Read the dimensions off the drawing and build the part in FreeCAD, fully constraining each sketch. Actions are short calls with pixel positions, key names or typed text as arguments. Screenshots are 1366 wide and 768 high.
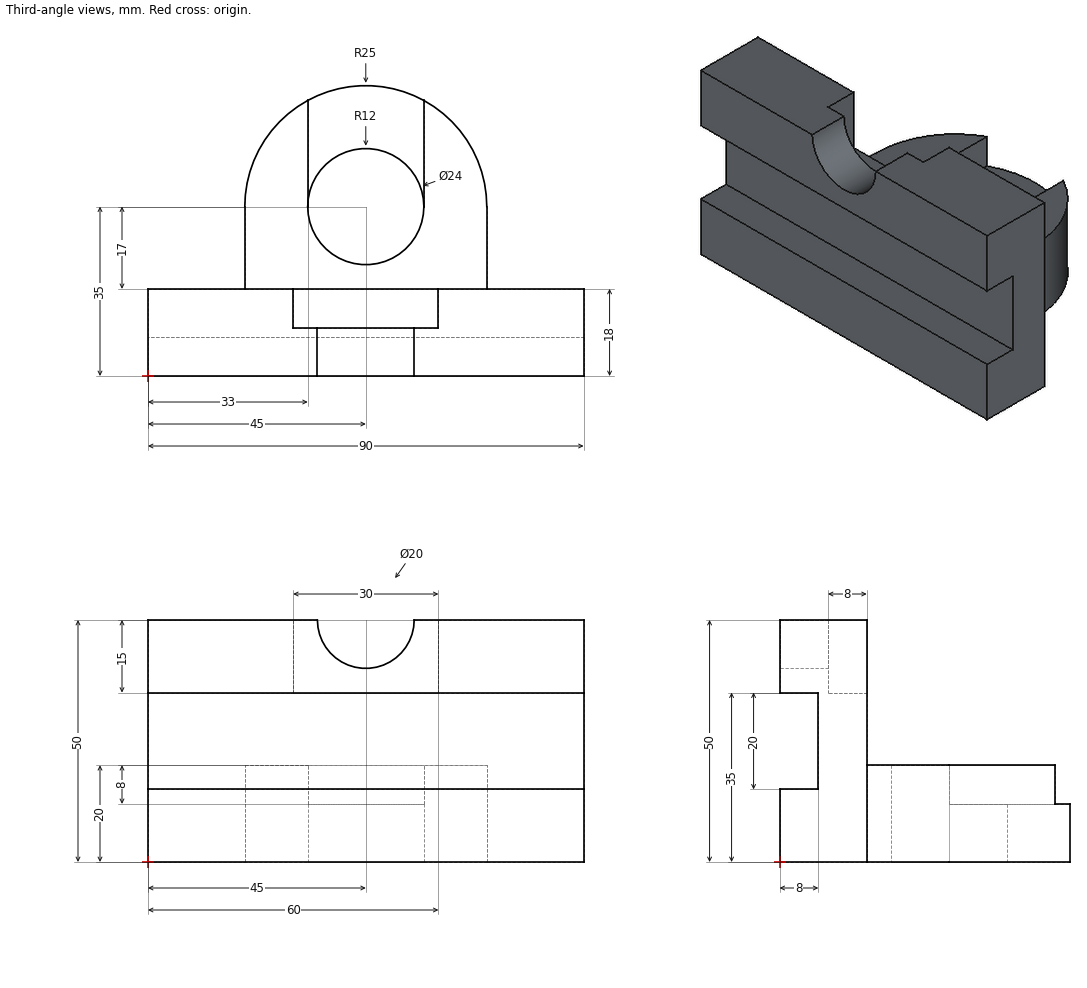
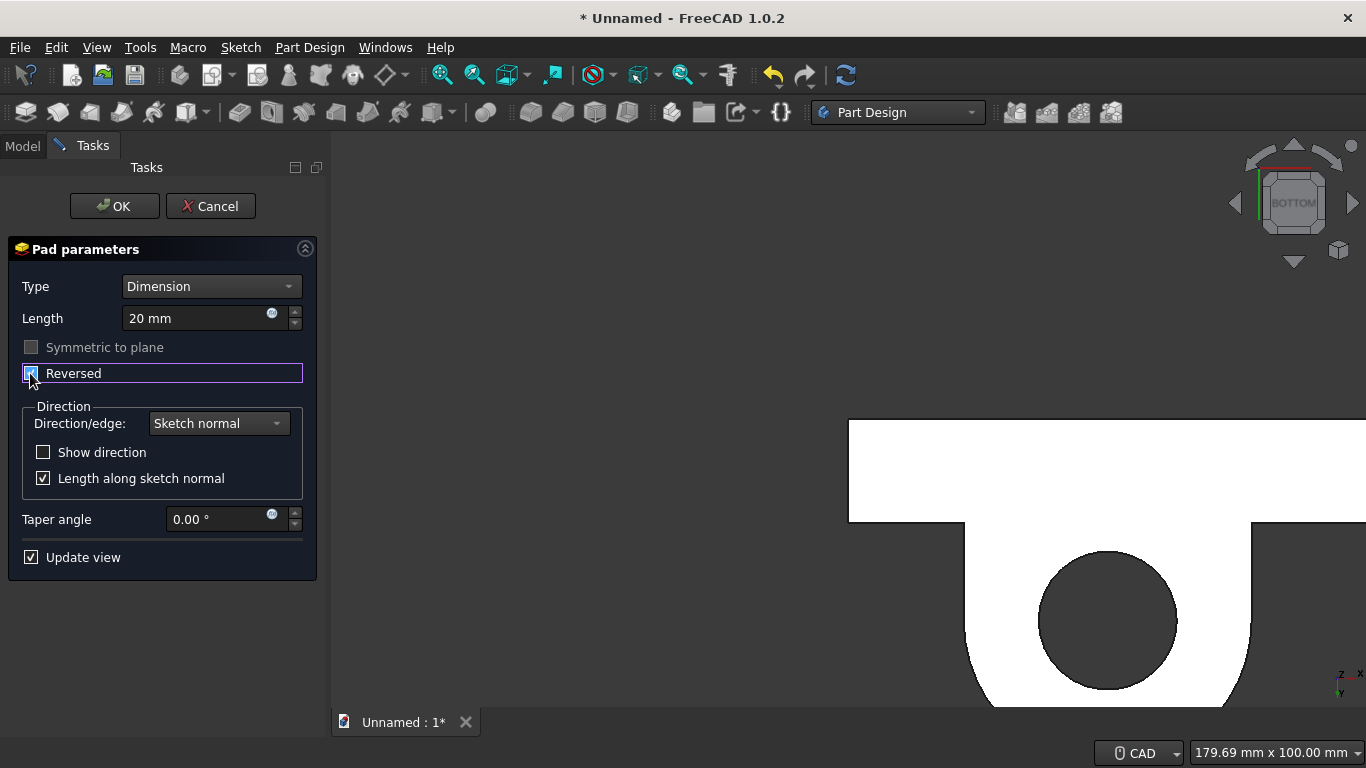
click(115, 206)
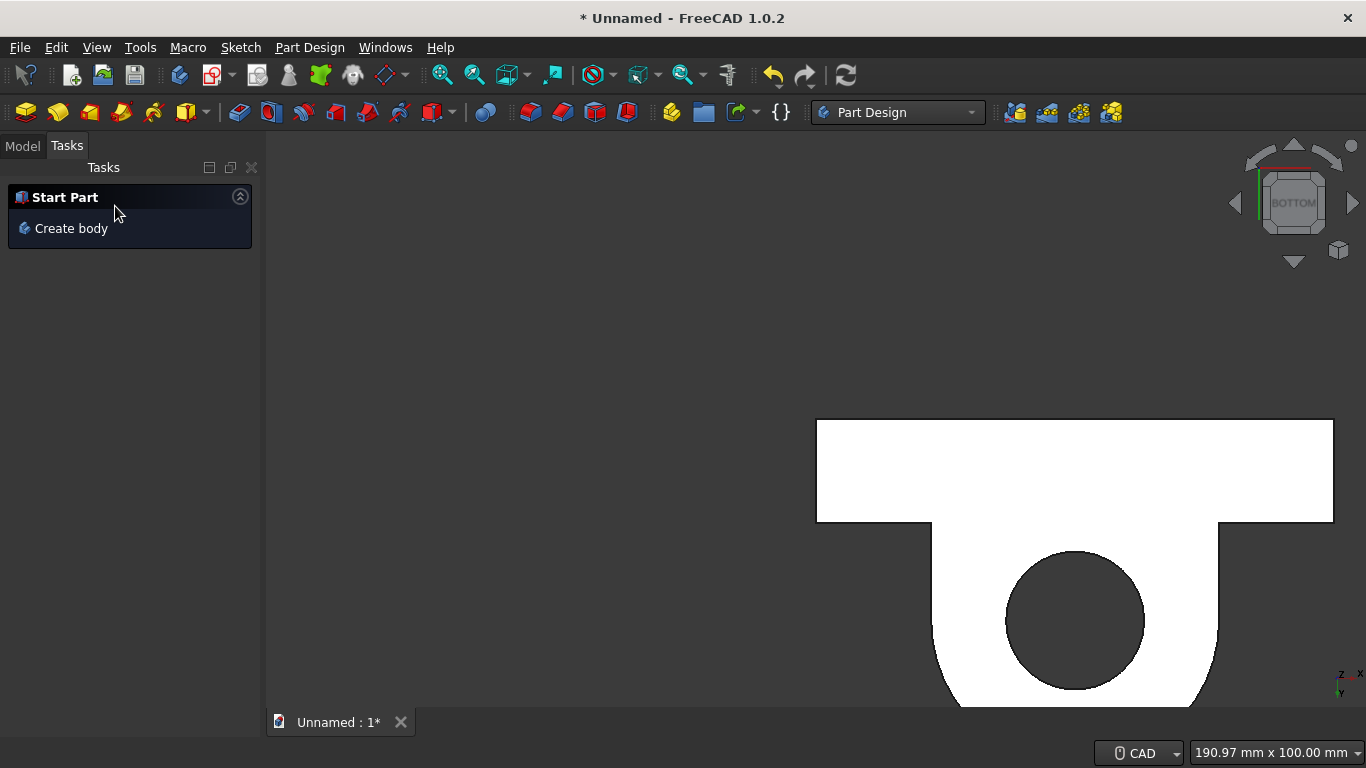
click(444, 76)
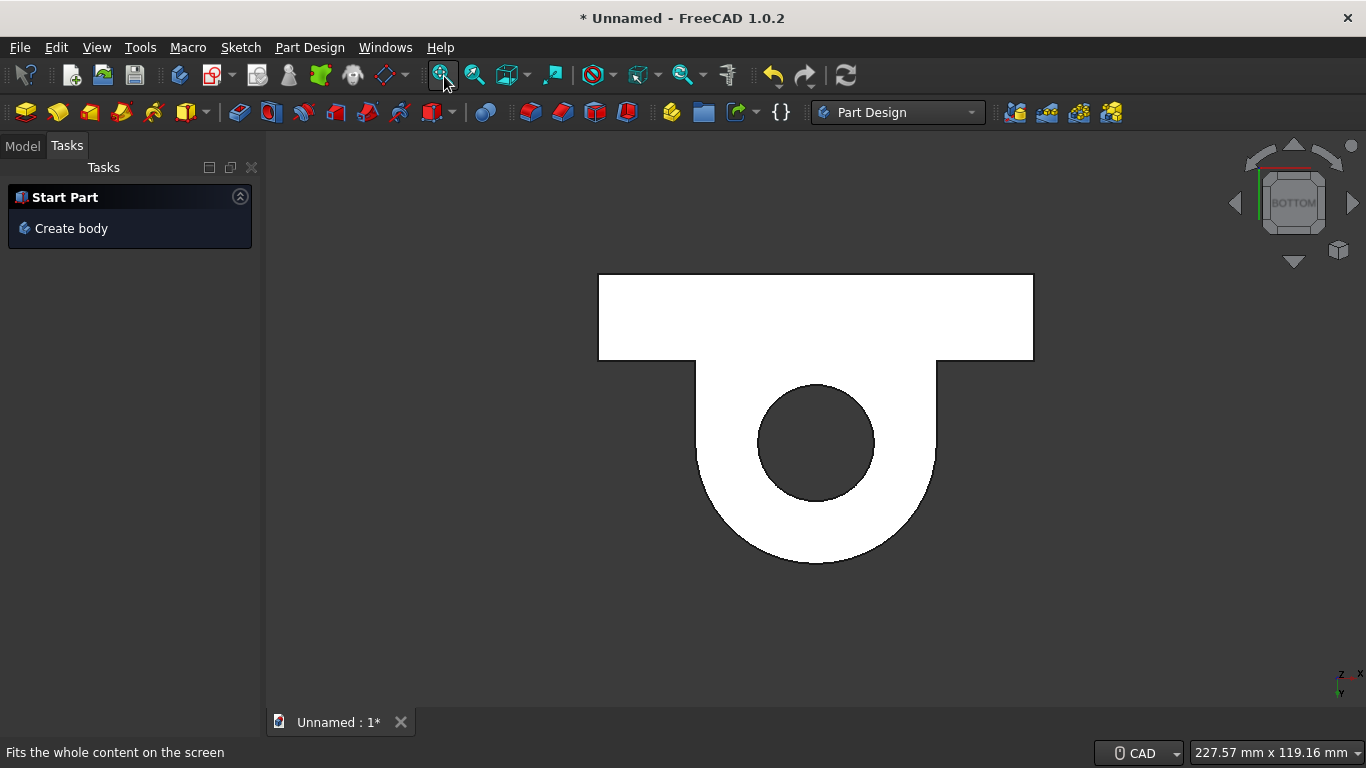
key(0)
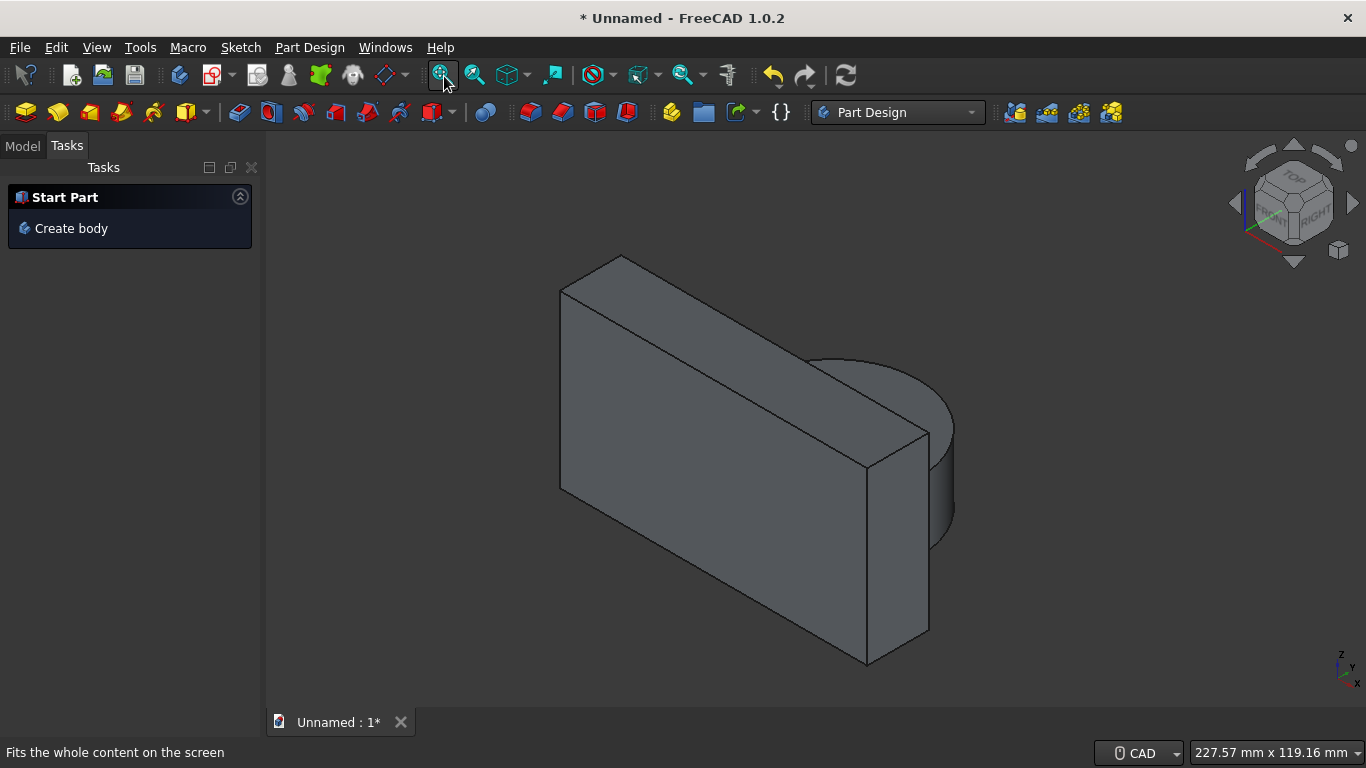
click(898, 492)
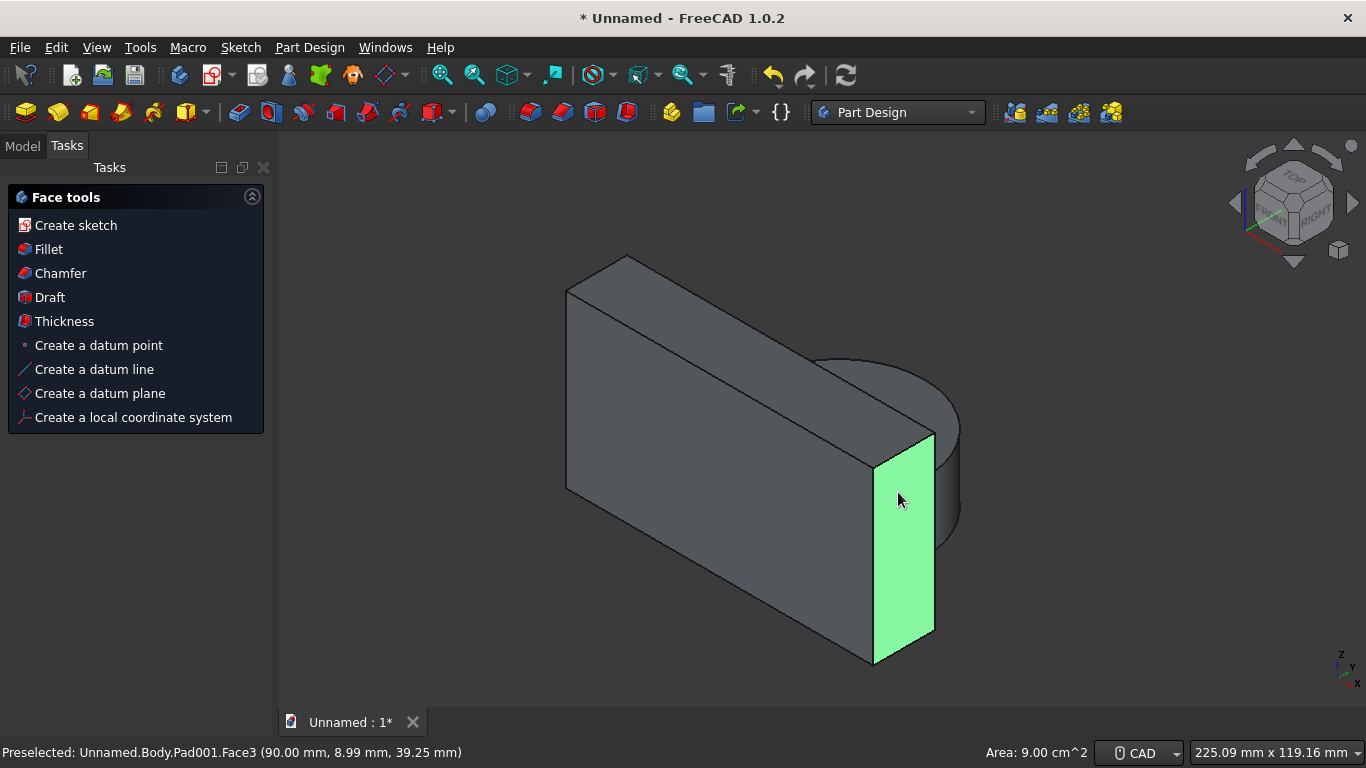
click(212, 76)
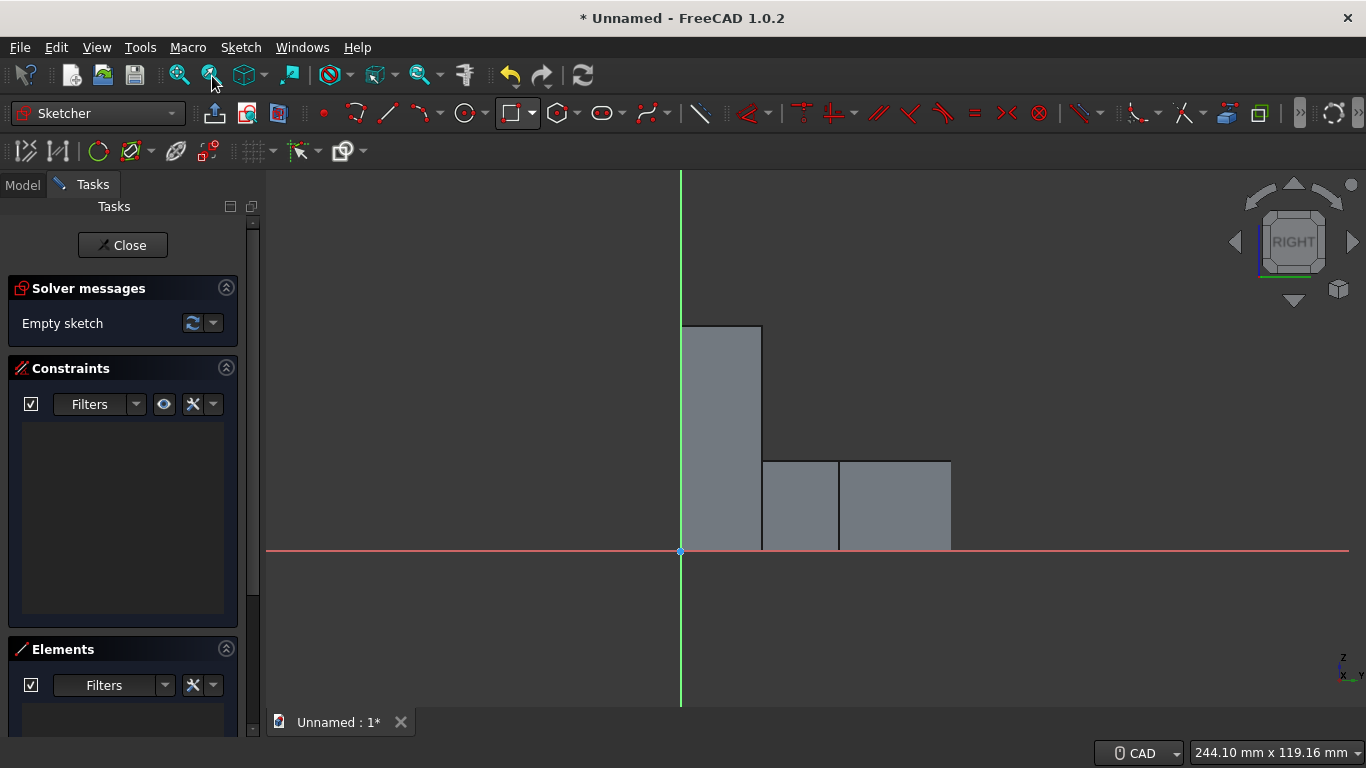
scroll(659, 500, up, 4)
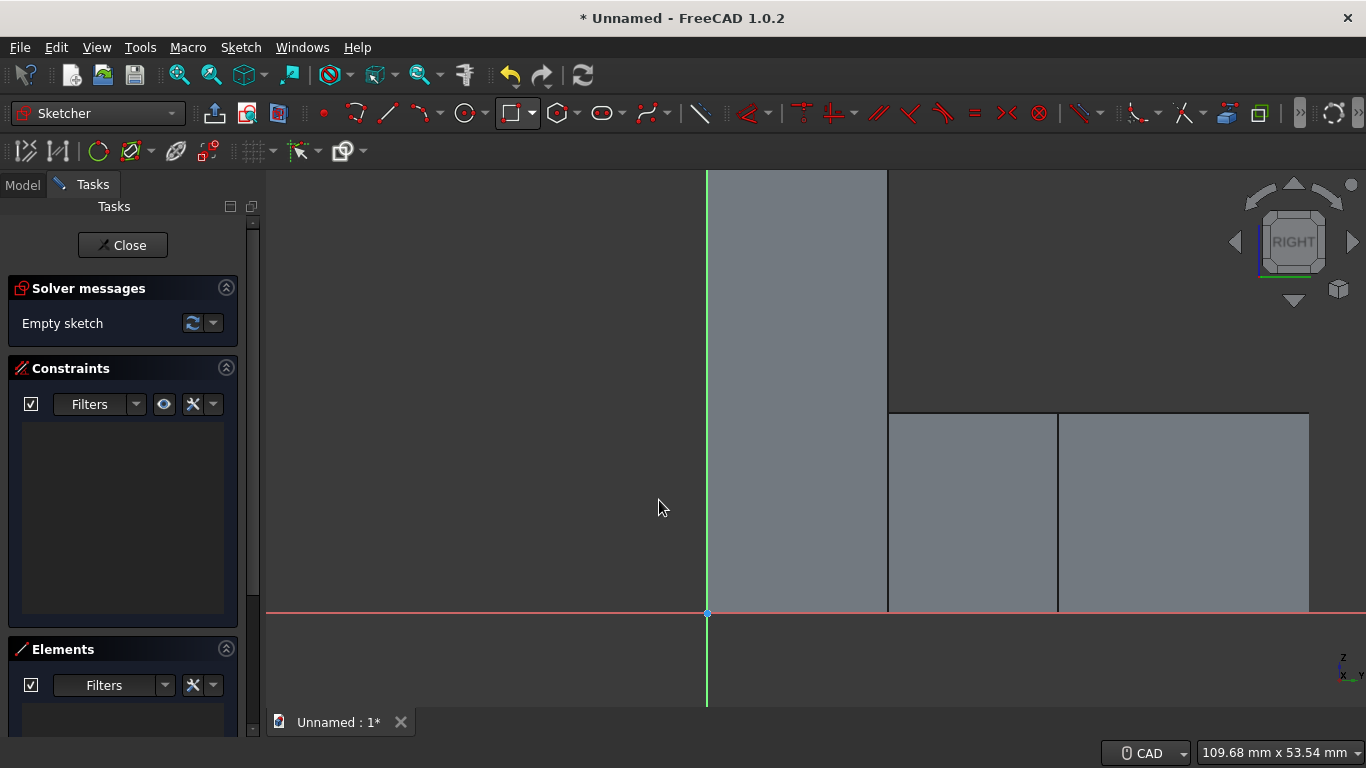
click(512, 114)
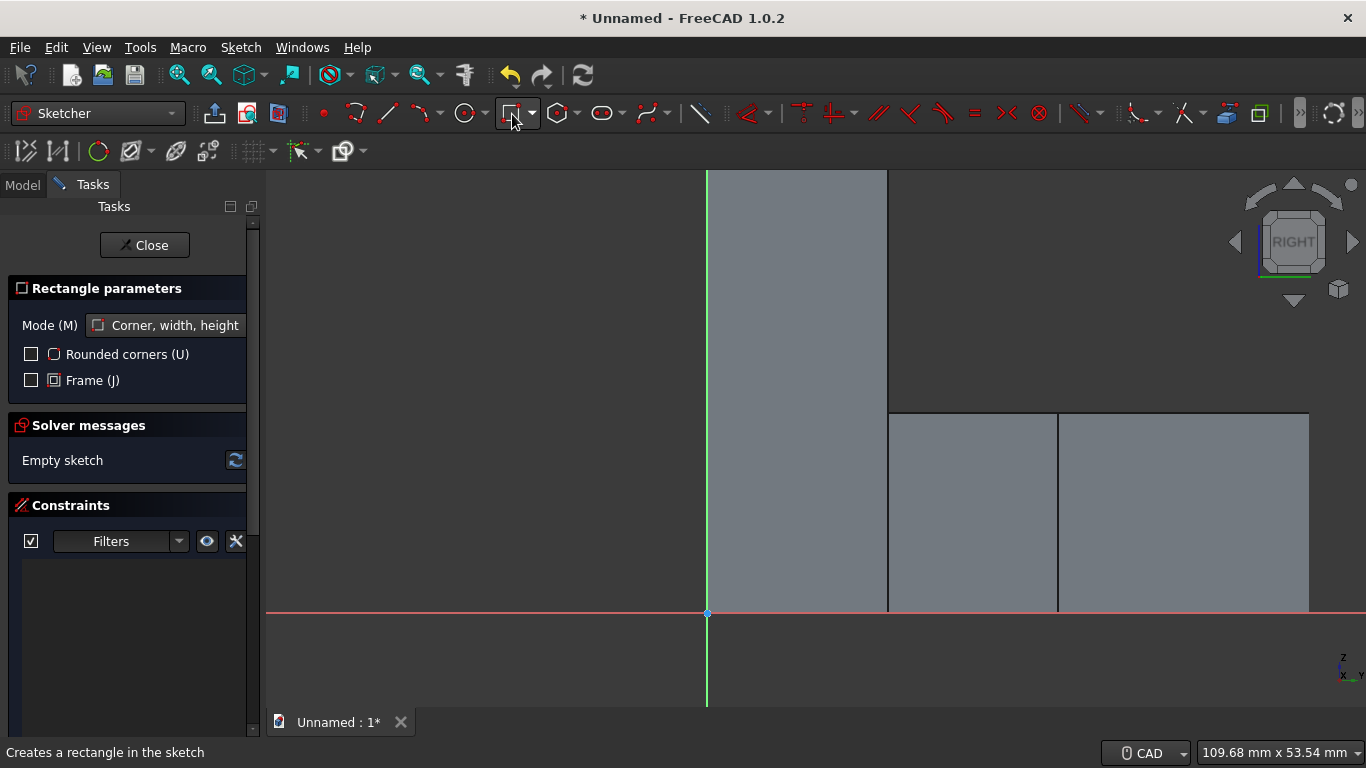
click(707, 262)
move(787, 463)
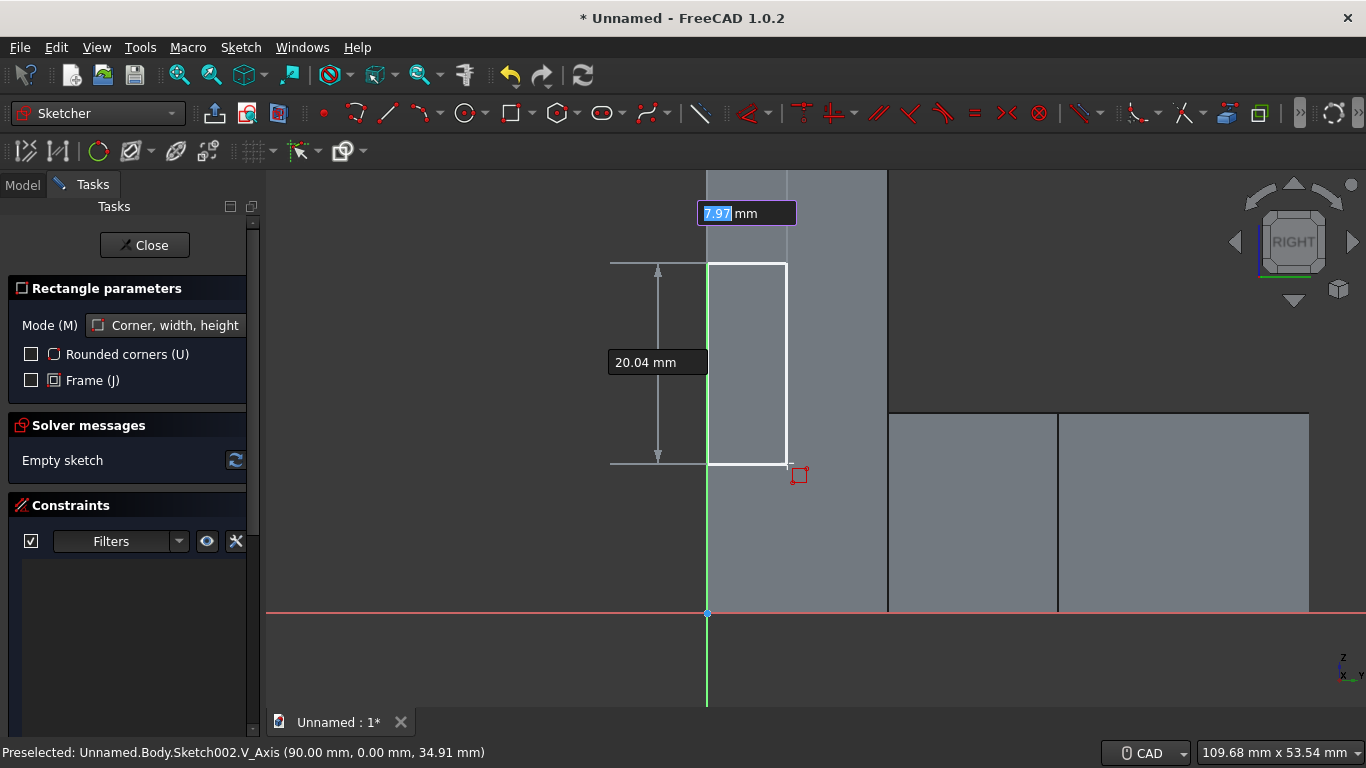
text(8)
key(Tab)
text(20)
key(Return)
key(Escape)